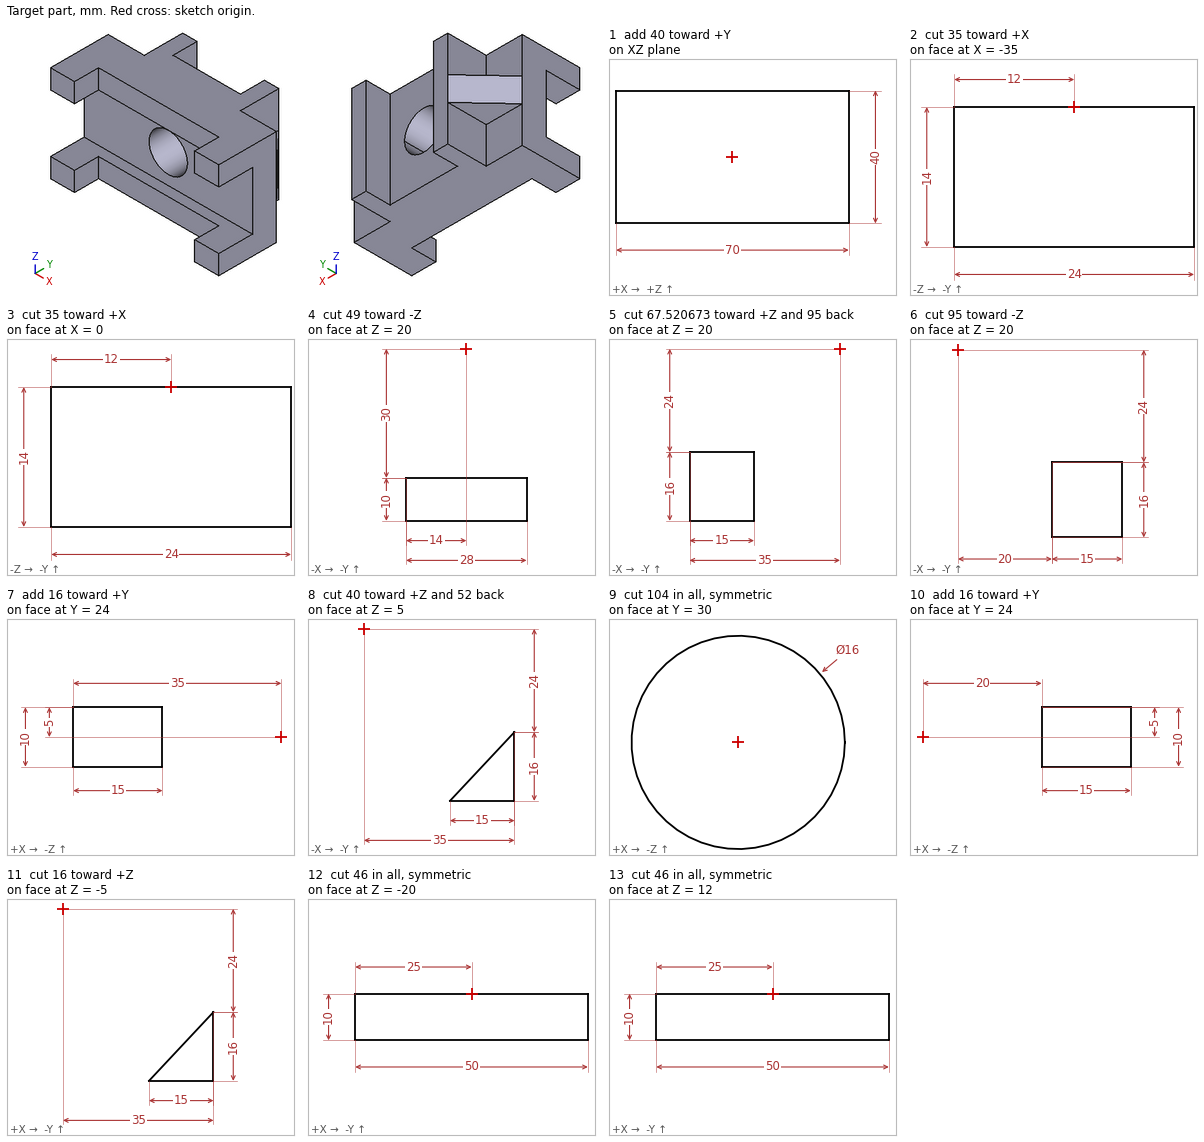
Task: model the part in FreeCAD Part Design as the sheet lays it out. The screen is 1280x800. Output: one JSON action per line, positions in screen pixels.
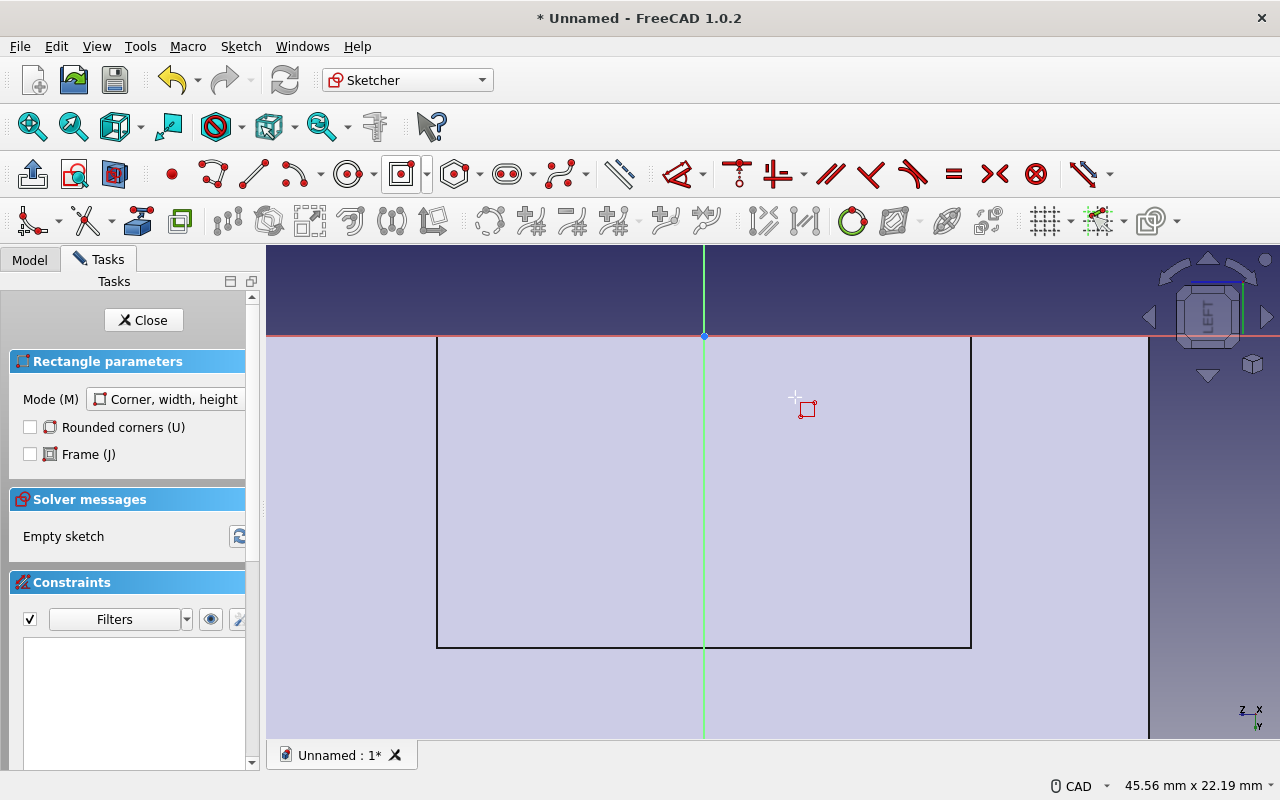
{"action": "left_click", "coordinate": [437, 336]}
{"action": "left_click", "coordinate": [971, 648]}
{"action": "key", "text": "Escape"}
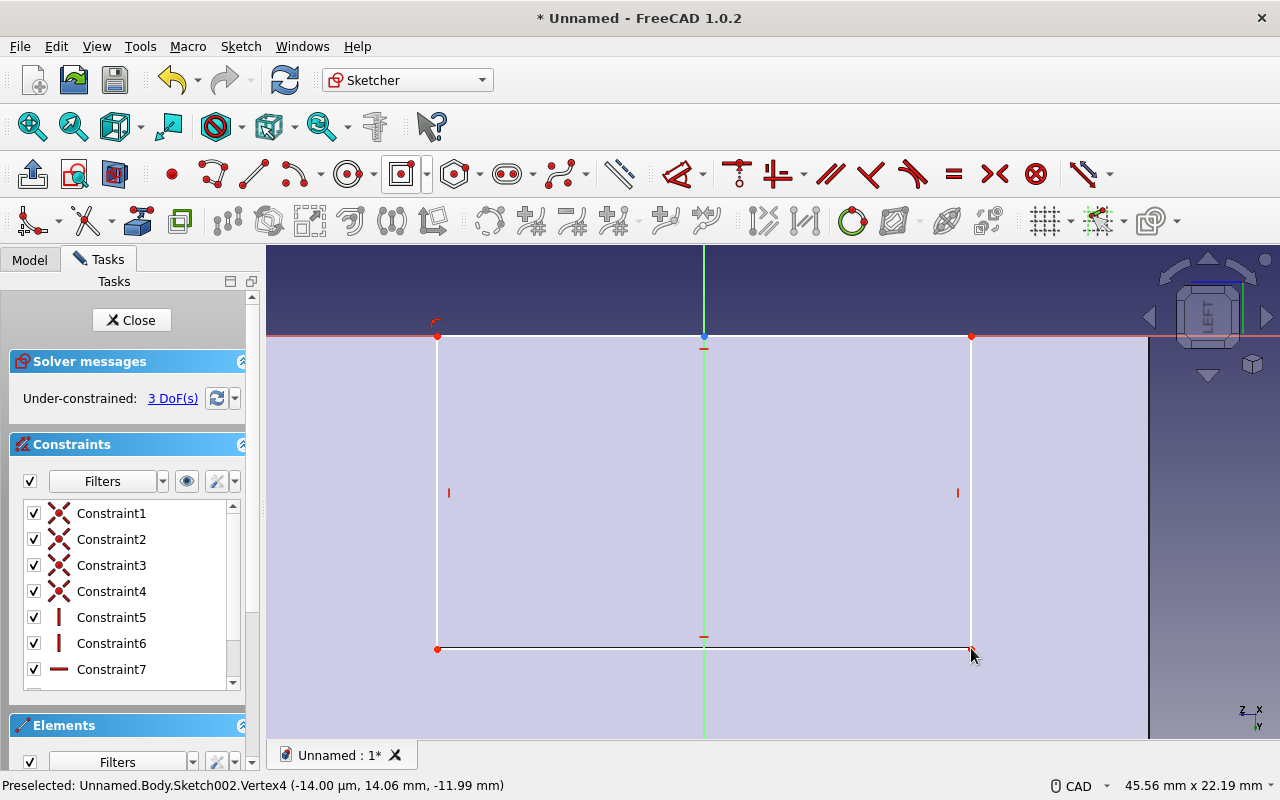
{"action": "left_click", "coordinate": [437, 430]}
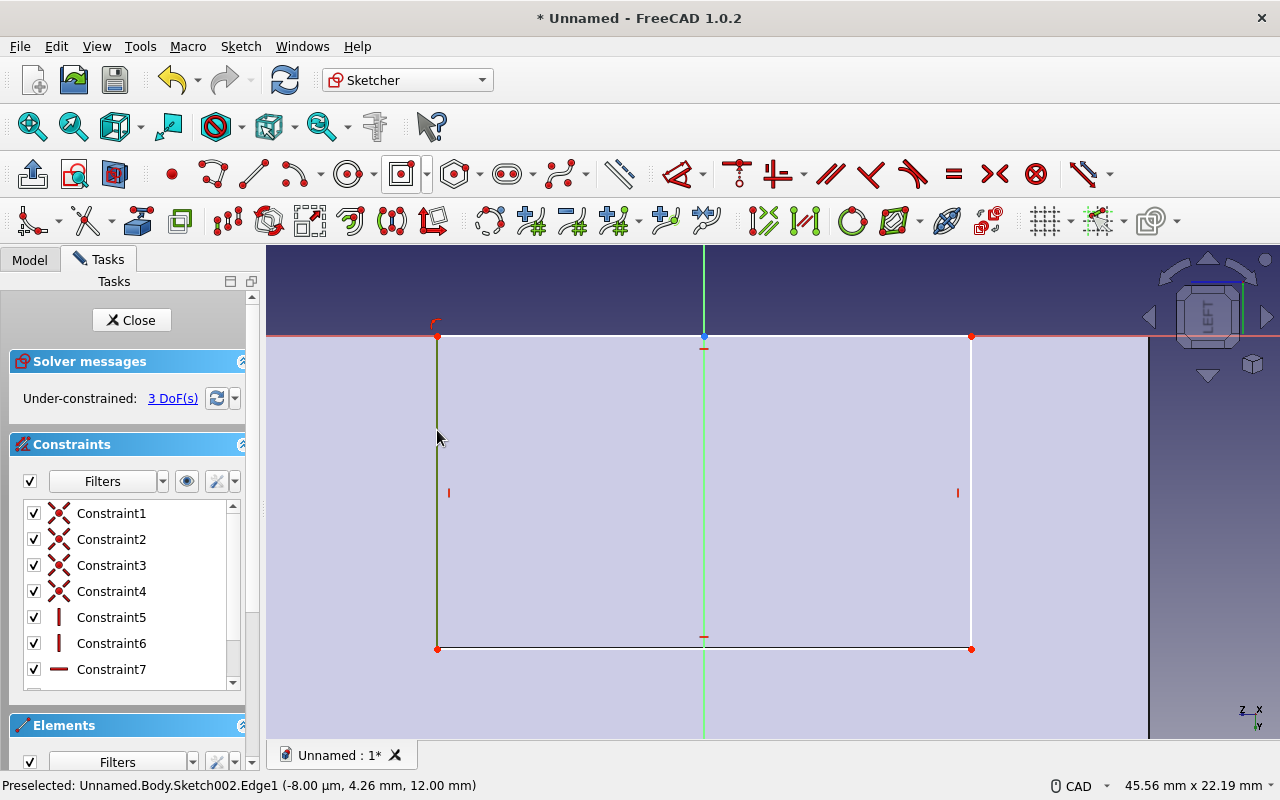
{"action": "left_click", "coordinate": [702, 174]}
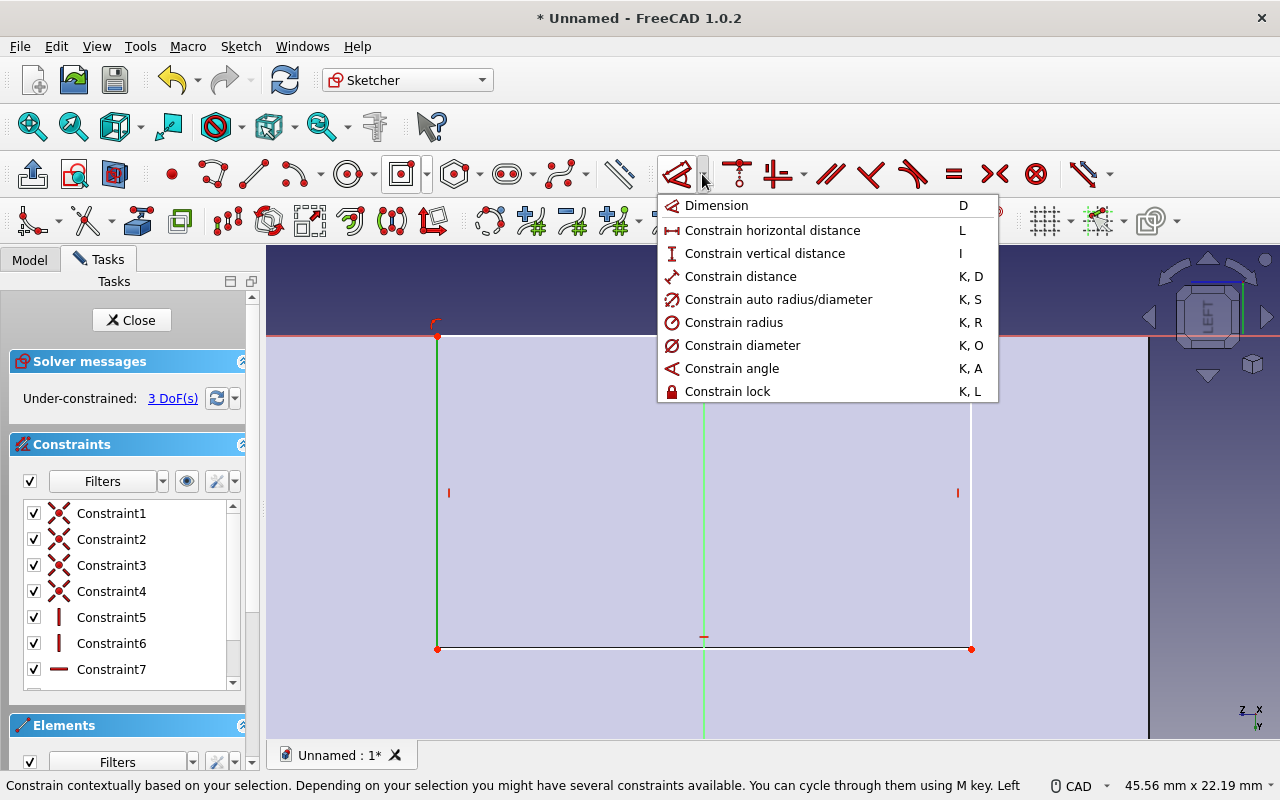
{"action": "left_click", "coordinate": [828, 254]}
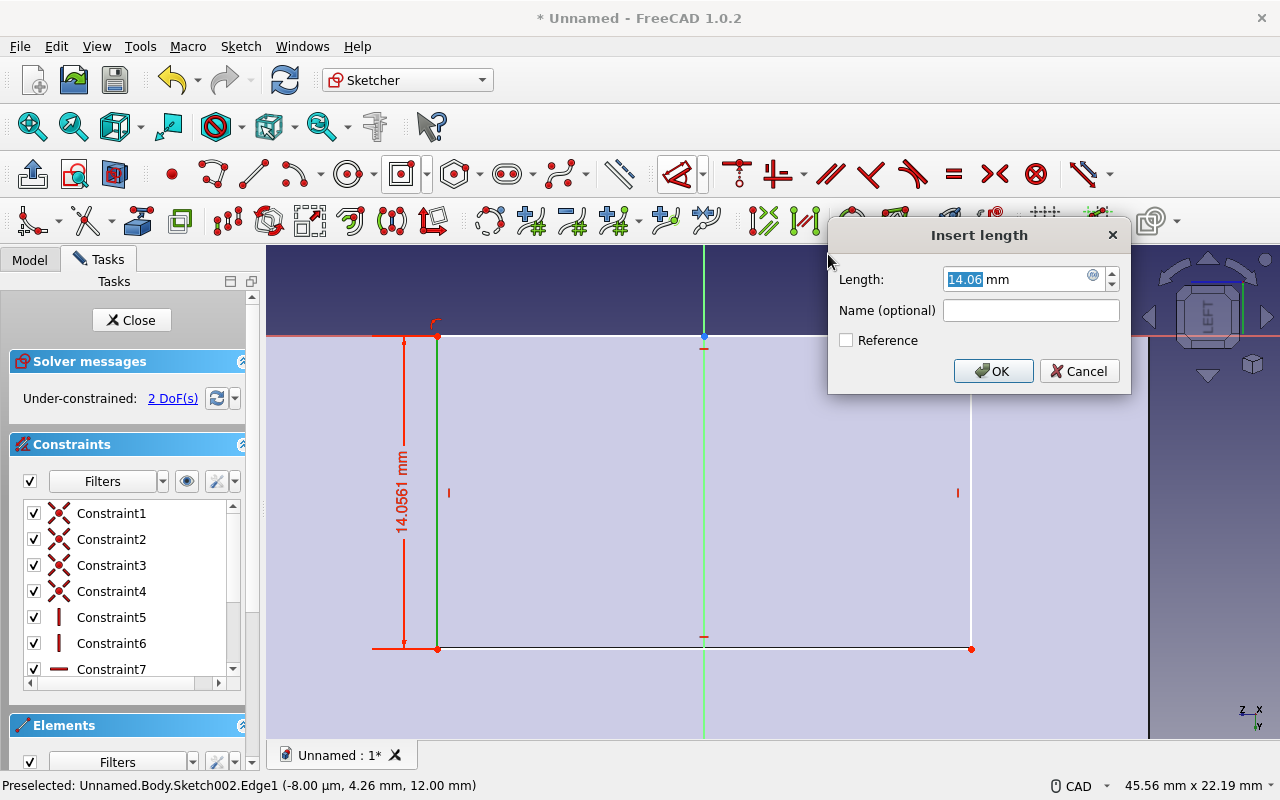
{"action": "type", "text": "14"}
{"action": "key", "text": "Return"}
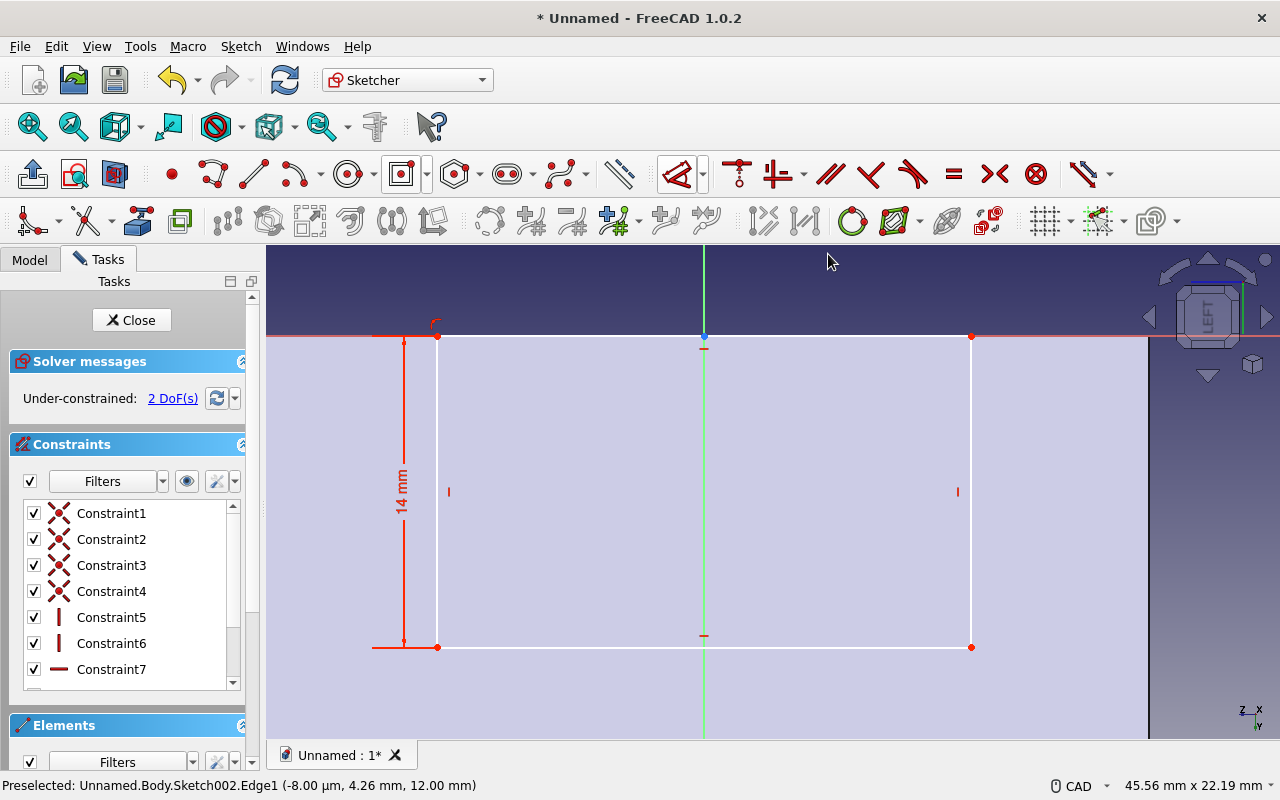
{"action": "left_click", "coordinate": [597, 648]}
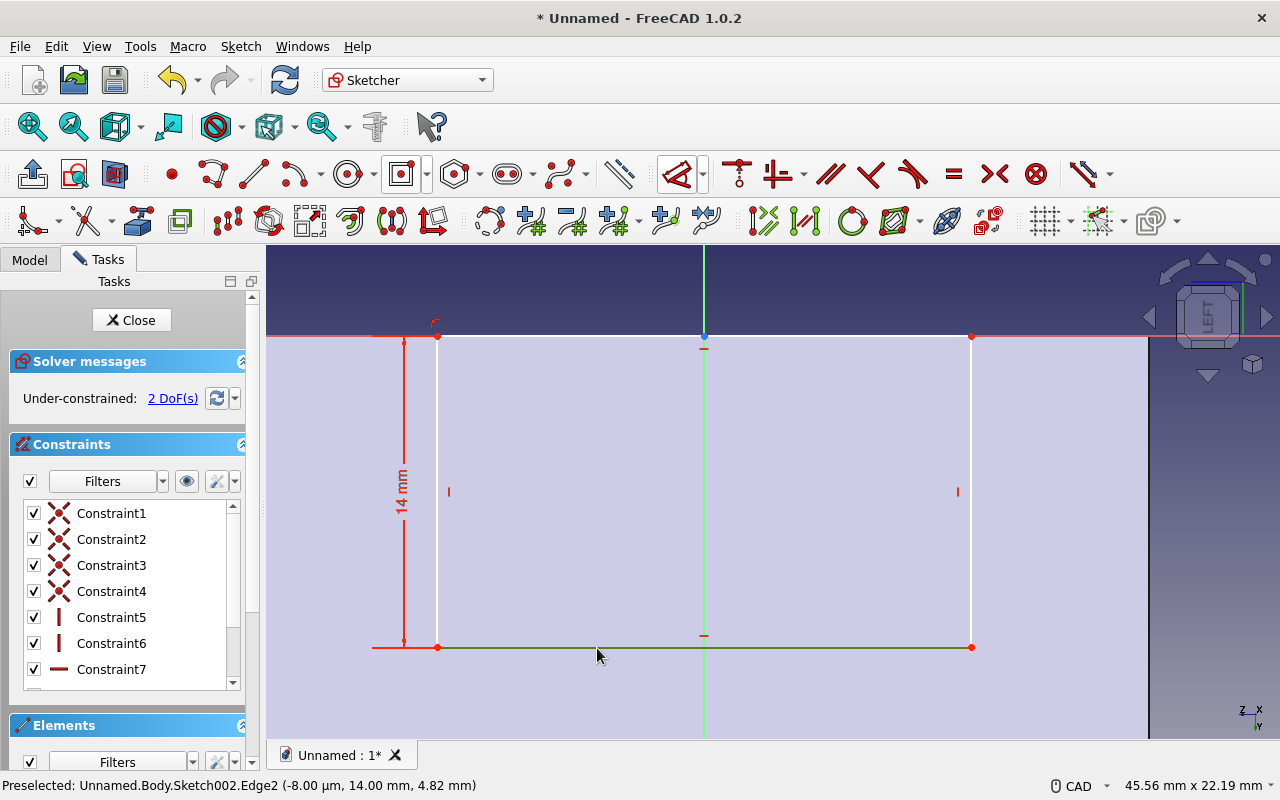
{"action": "left_click", "coordinate": [702, 174]}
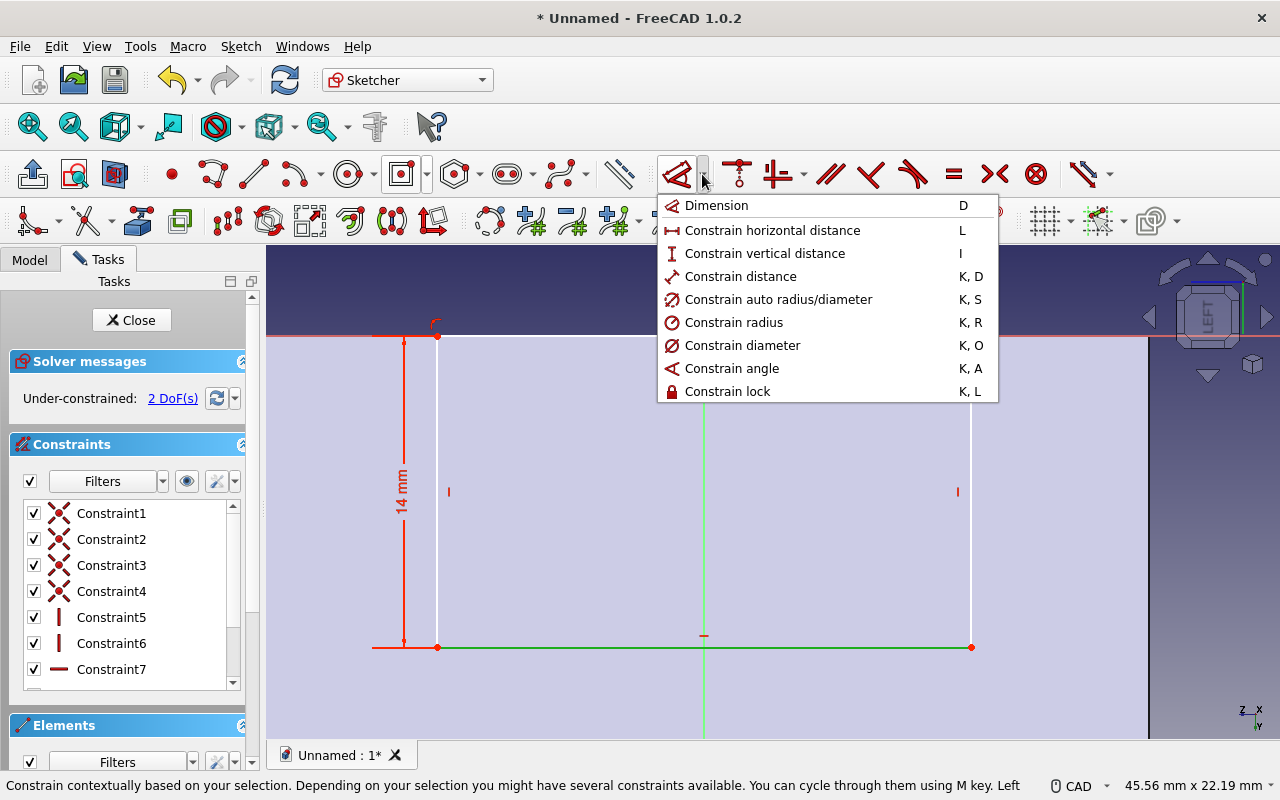
{"action": "left_click", "coordinate": [828, 230]}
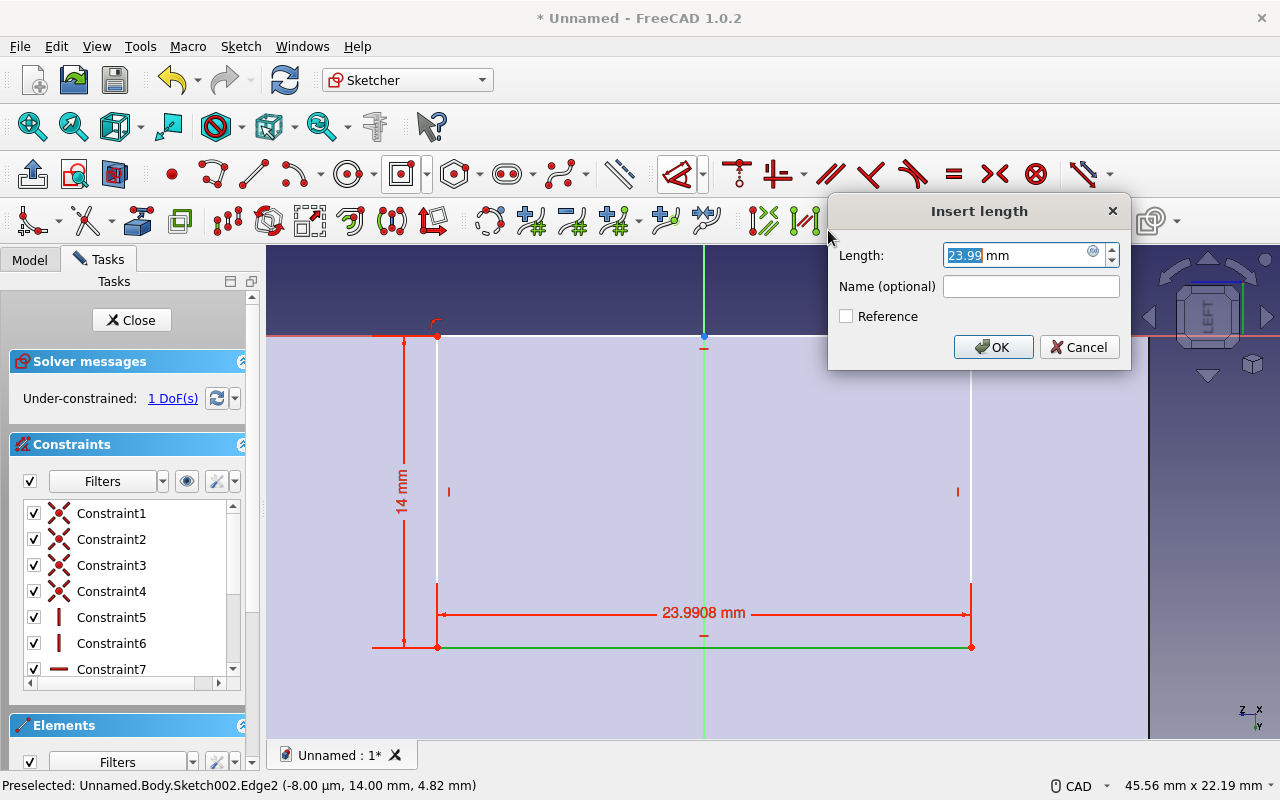
{"action": "type", "text": "24"}
{"action": "key", "text": "Return"}